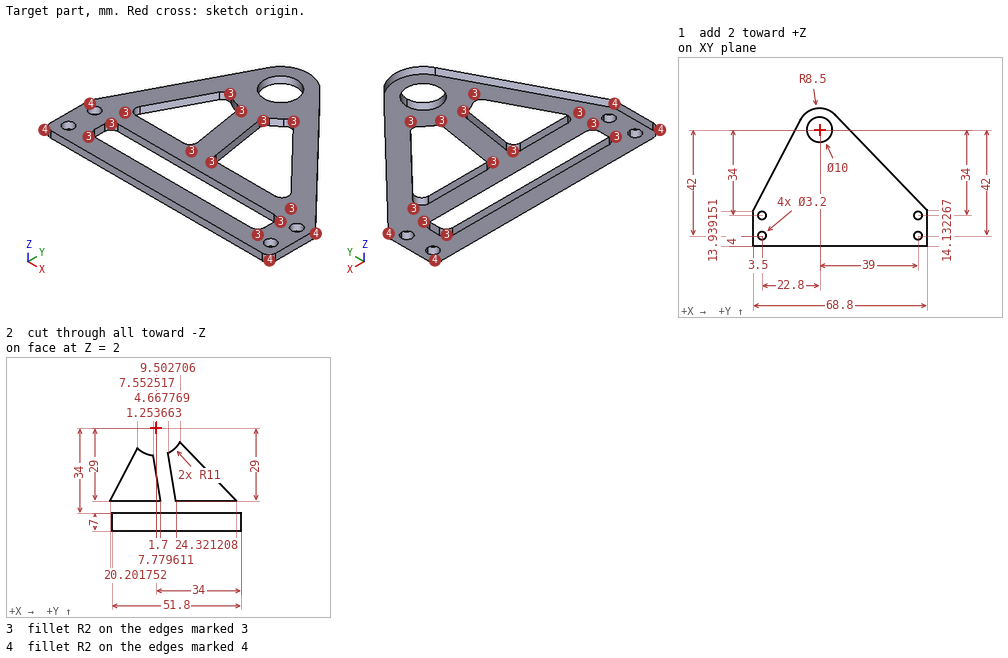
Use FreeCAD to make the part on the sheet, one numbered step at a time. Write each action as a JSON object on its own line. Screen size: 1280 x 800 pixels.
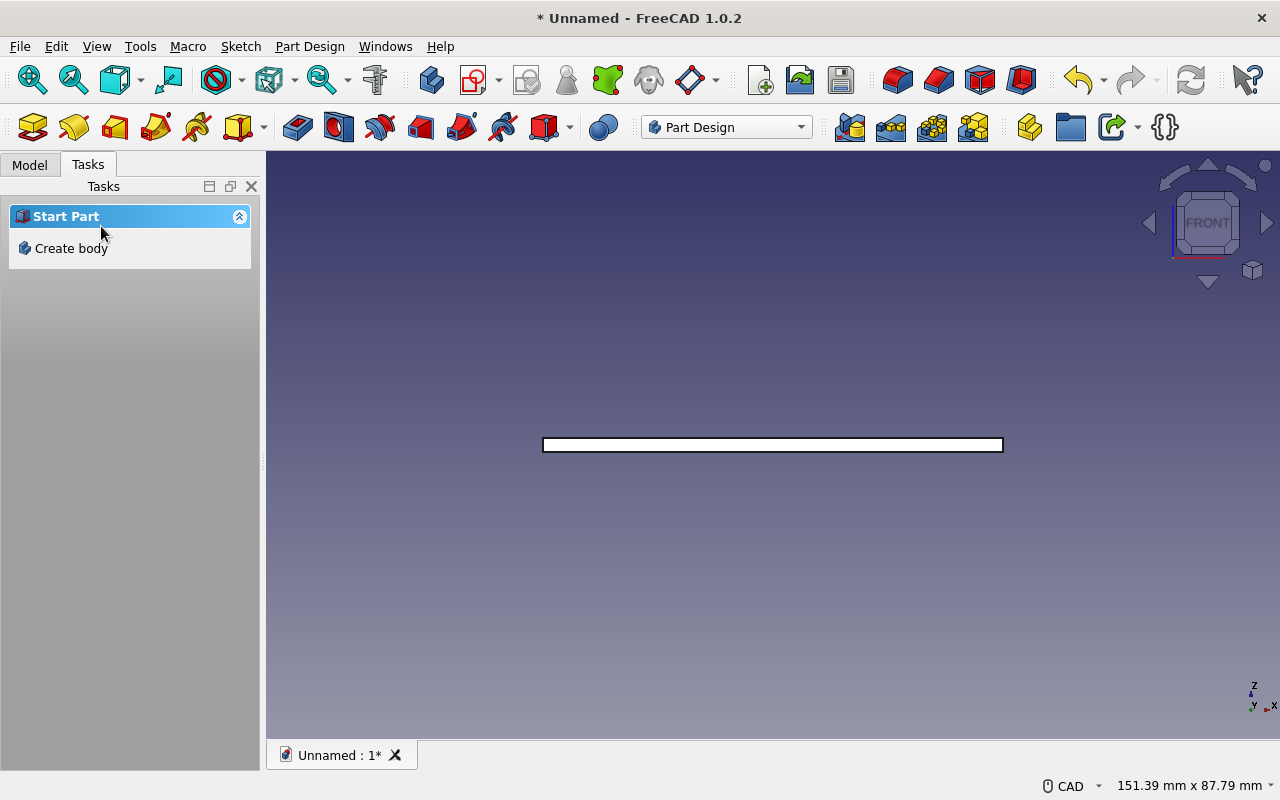
{"action": "left_click", "coordinate": [1003, 444]}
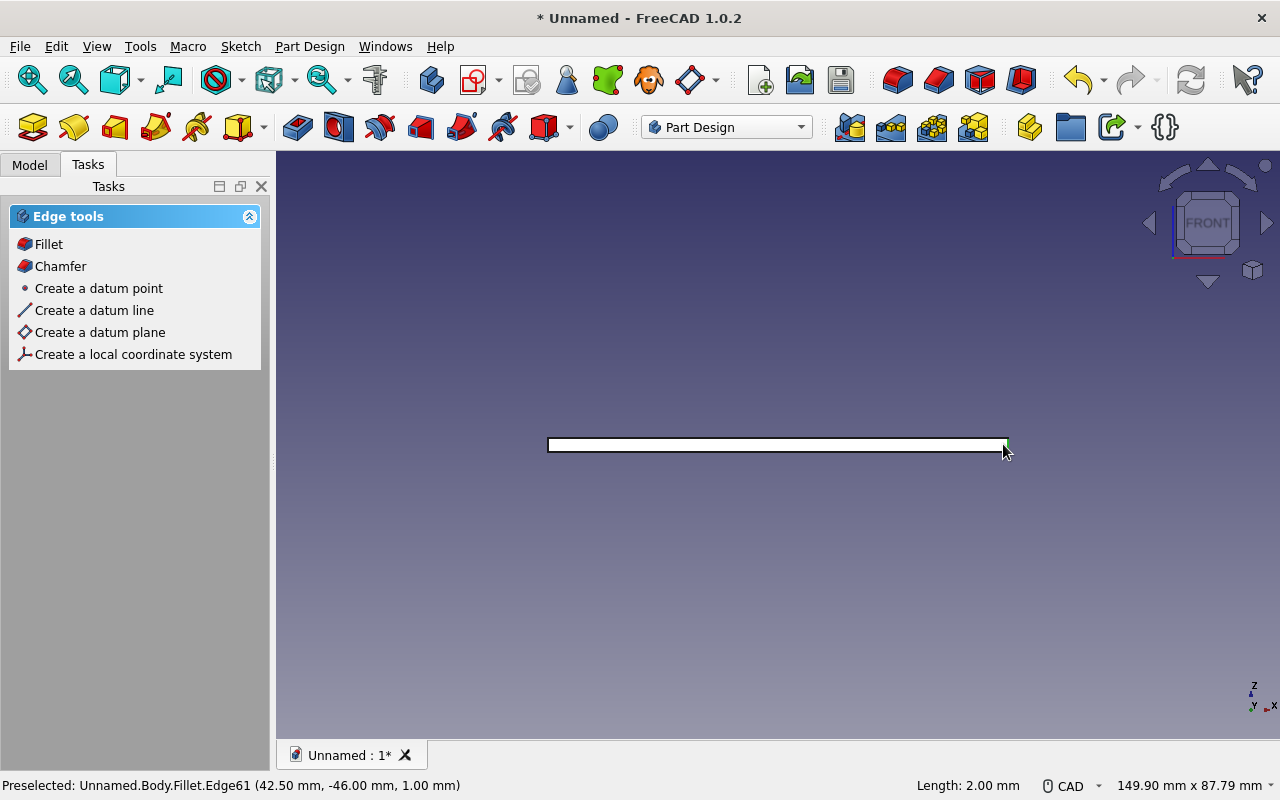
{"action": "left_click", "coordinate": [548, 444], "text": "ctrl"}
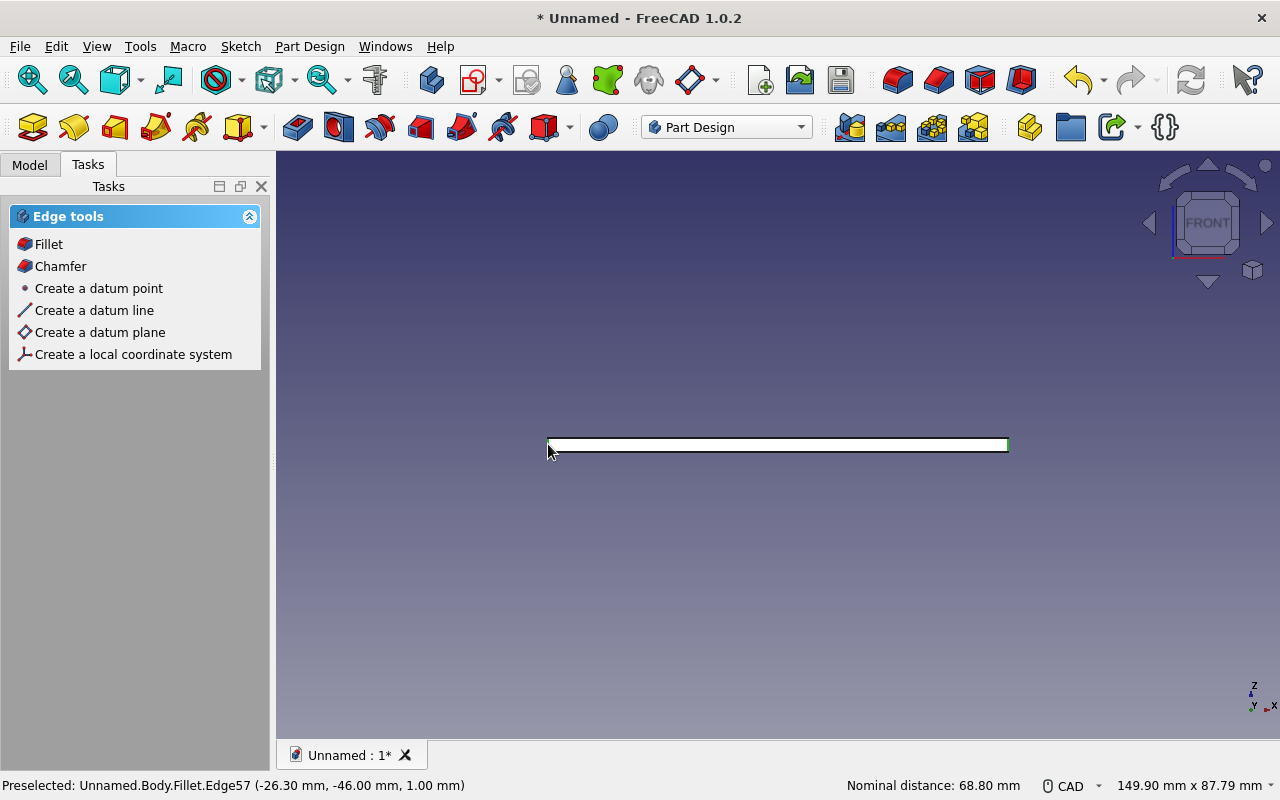
{"action": "scroll", "coordinate": [1008, 444], "scroll_direction": "up", "scroll_amount": 6}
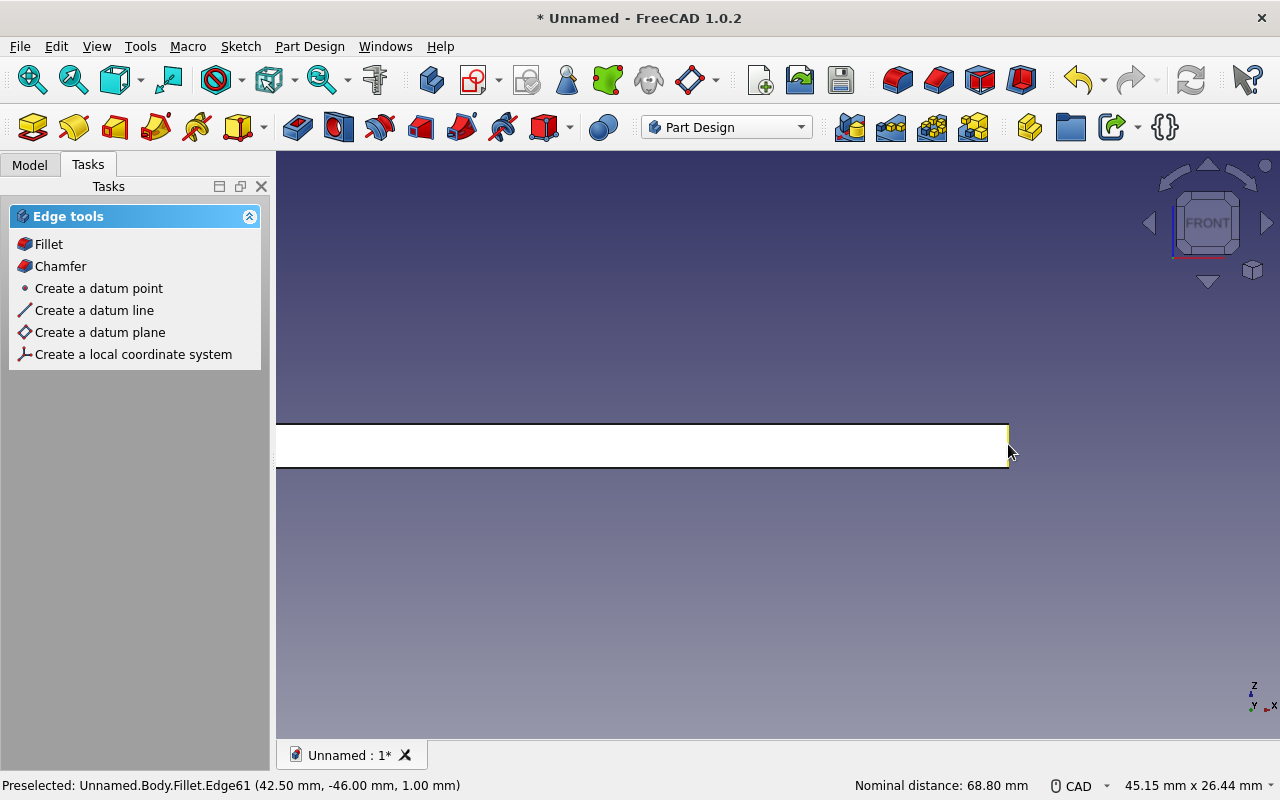
{"action": "left_click", "coordinate": [33, 80]}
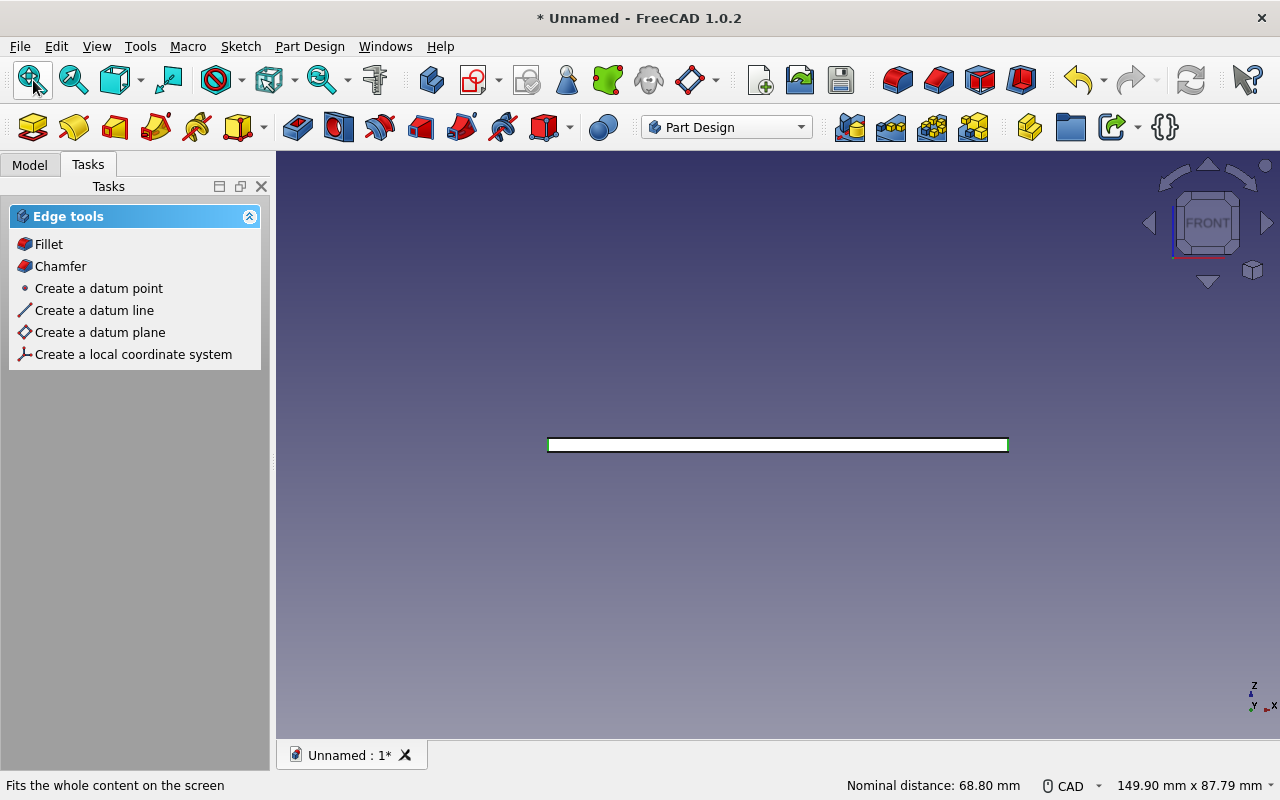
{"action": "key", "text": "0"}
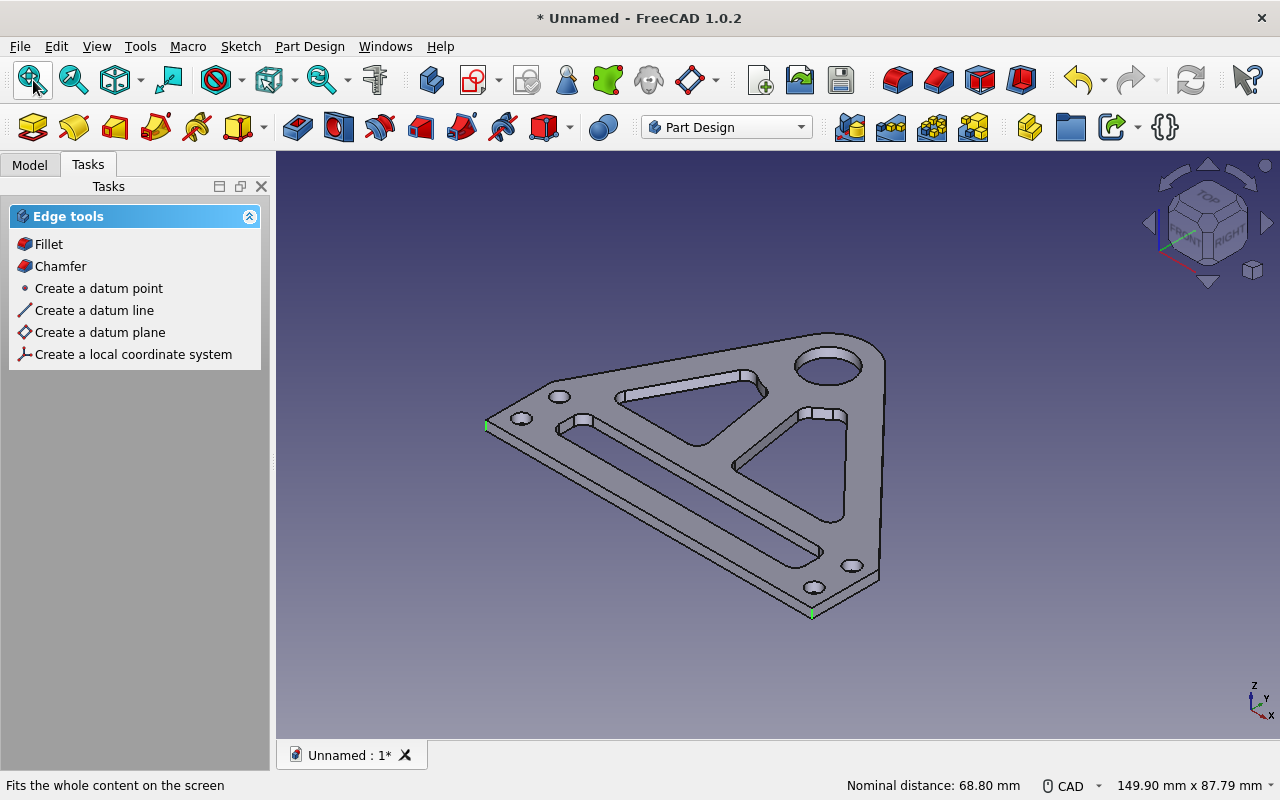
{"action": "scroll", "coordinate": [879, 574], "scroll_direction": "up", "scroll_amount": 6}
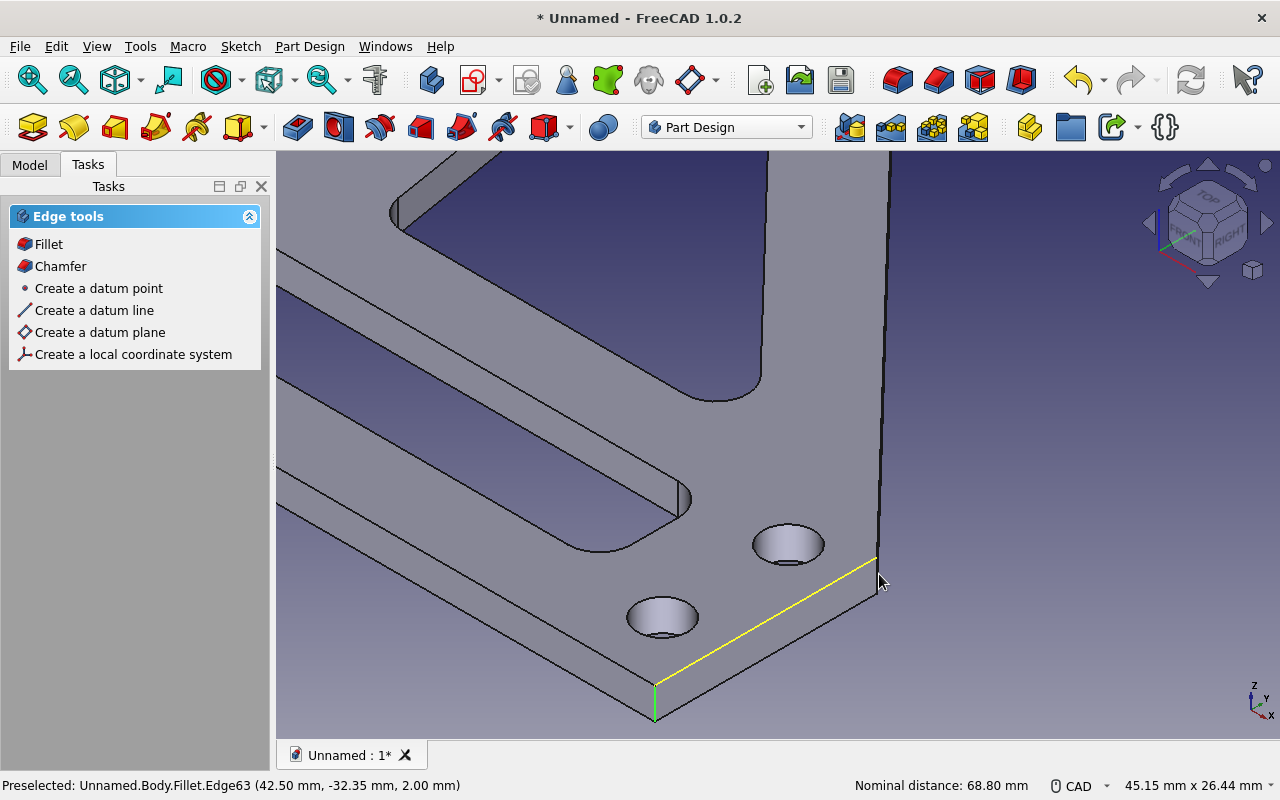
{"action": "left_click", "coordinate": [33, 80]}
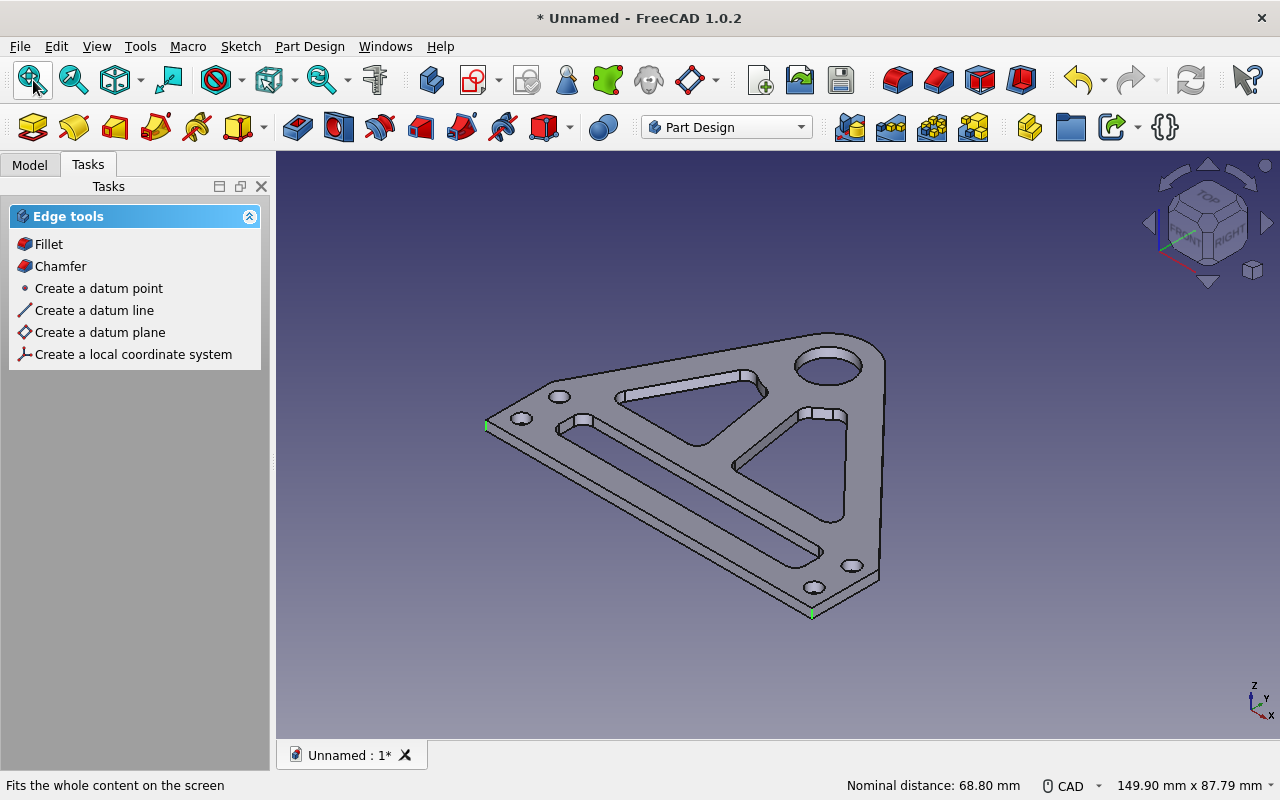
{"action": "key", "text": "2"}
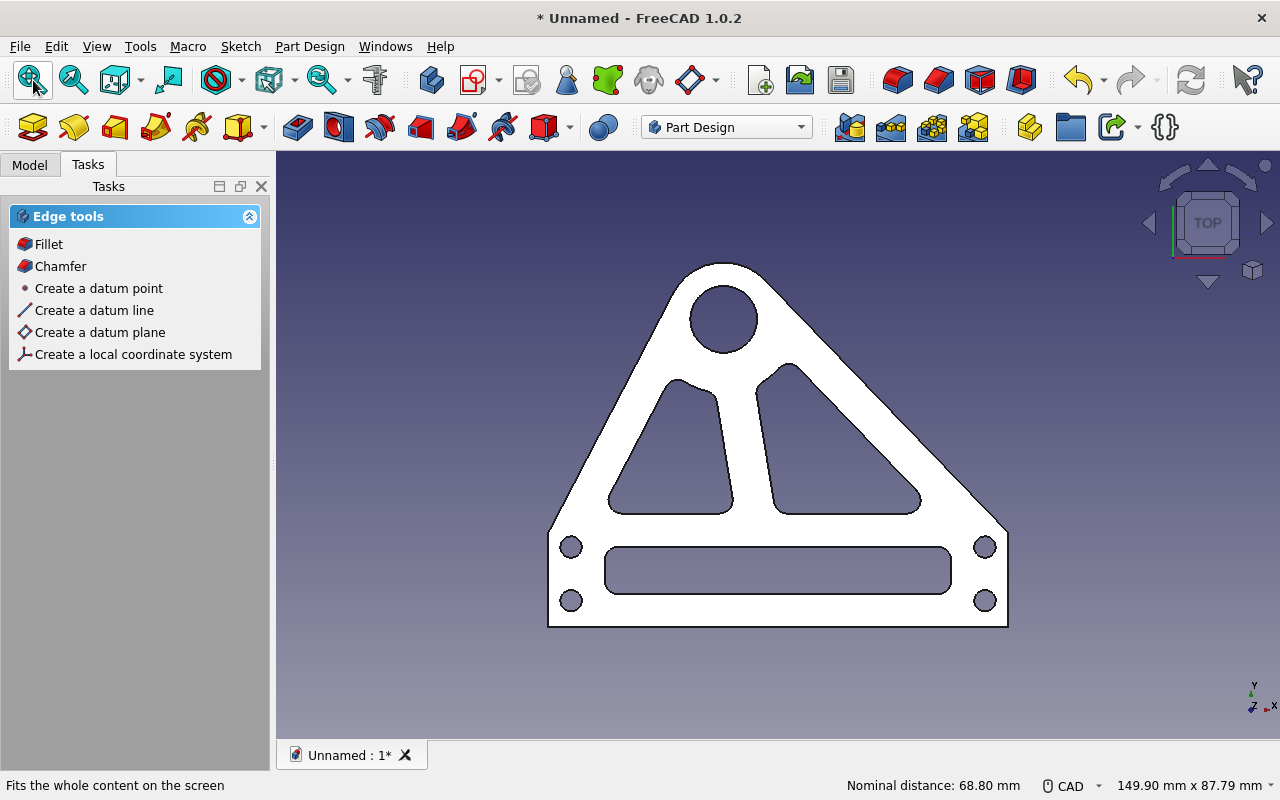
{"action": "scroll", "coordinate": [1008, 532], "scroll_direction": "up", "scroll_amount": 6}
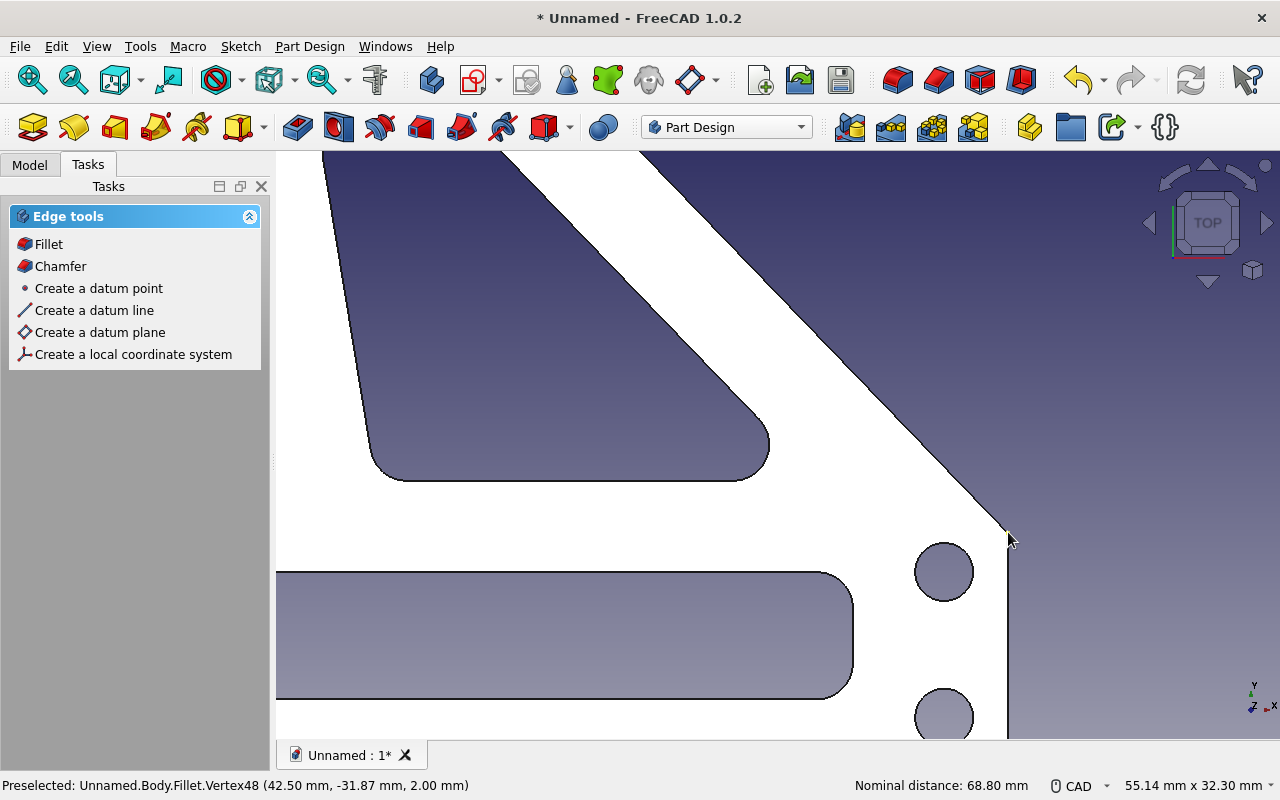
{"action": "key", "text": "v f"}